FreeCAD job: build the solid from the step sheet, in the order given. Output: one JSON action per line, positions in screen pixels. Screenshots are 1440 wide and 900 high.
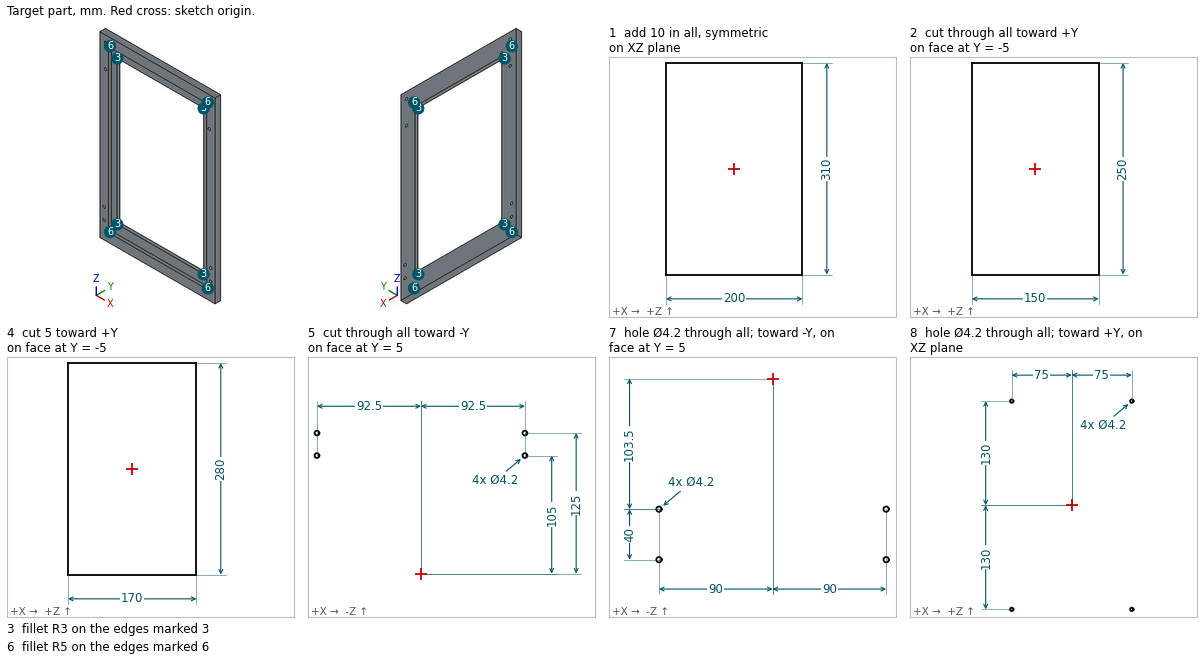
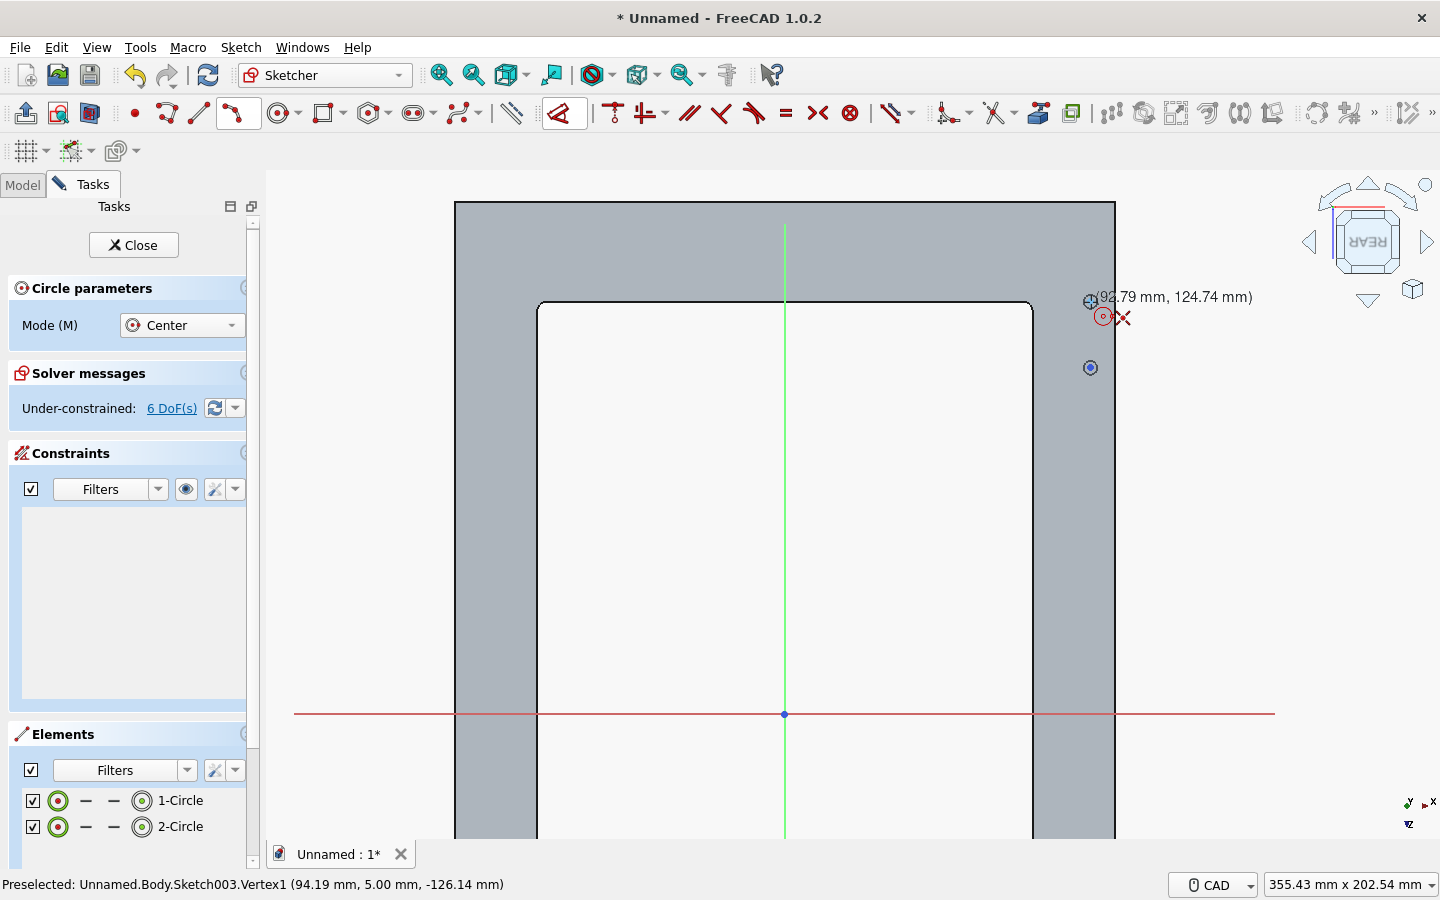
{"action": "scroll", "coordinate": [479, 368], "scroll_direction": "up", "scroll_amount": 6}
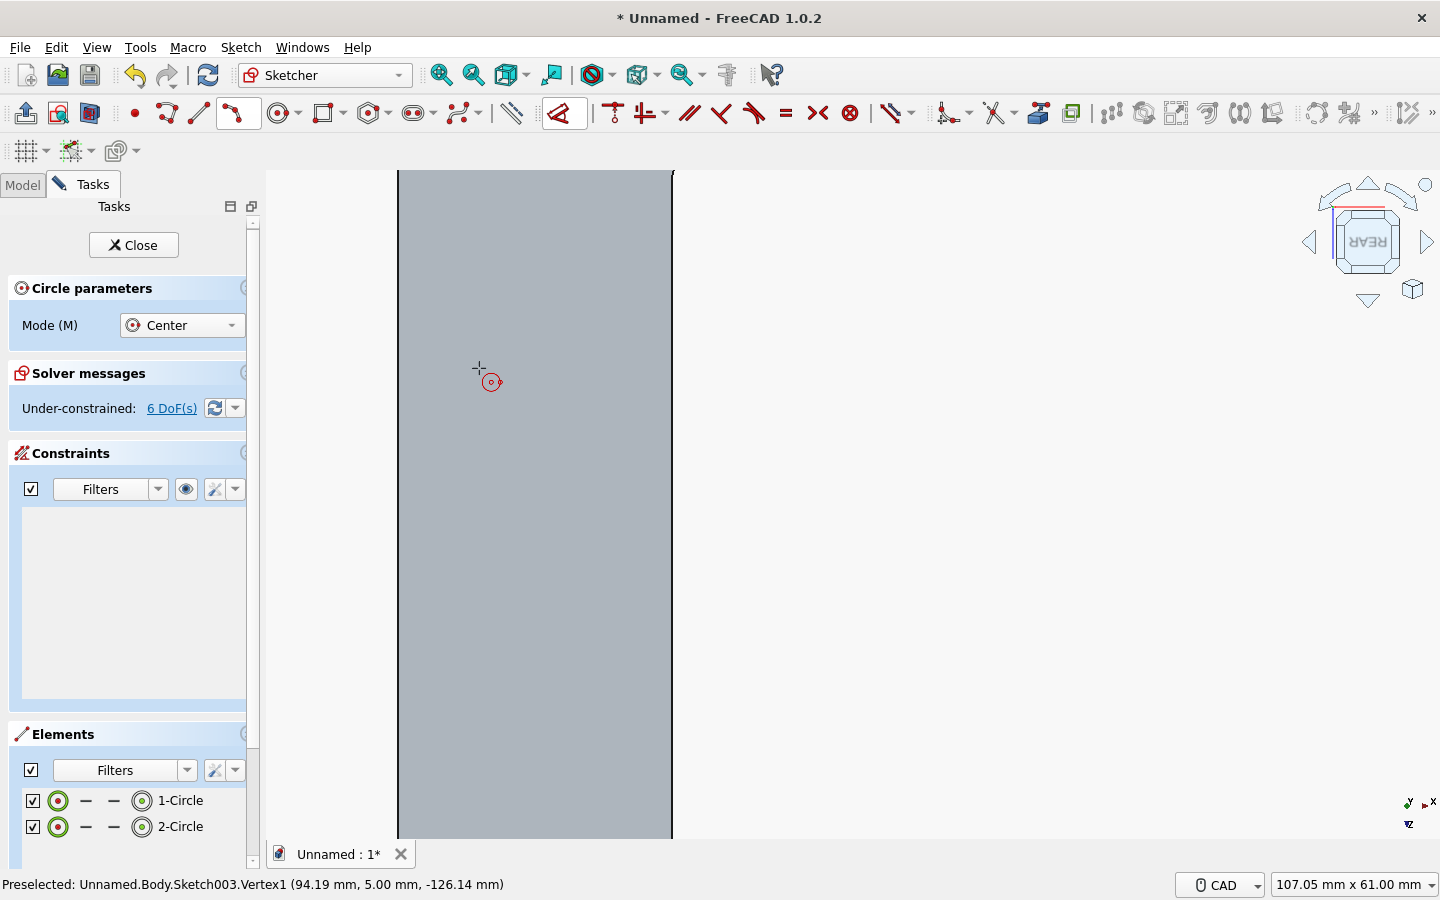
{"action": "left_click", "coordinate": [480, 366]}
{"action": "left_click", "coordinate": [496, 350]}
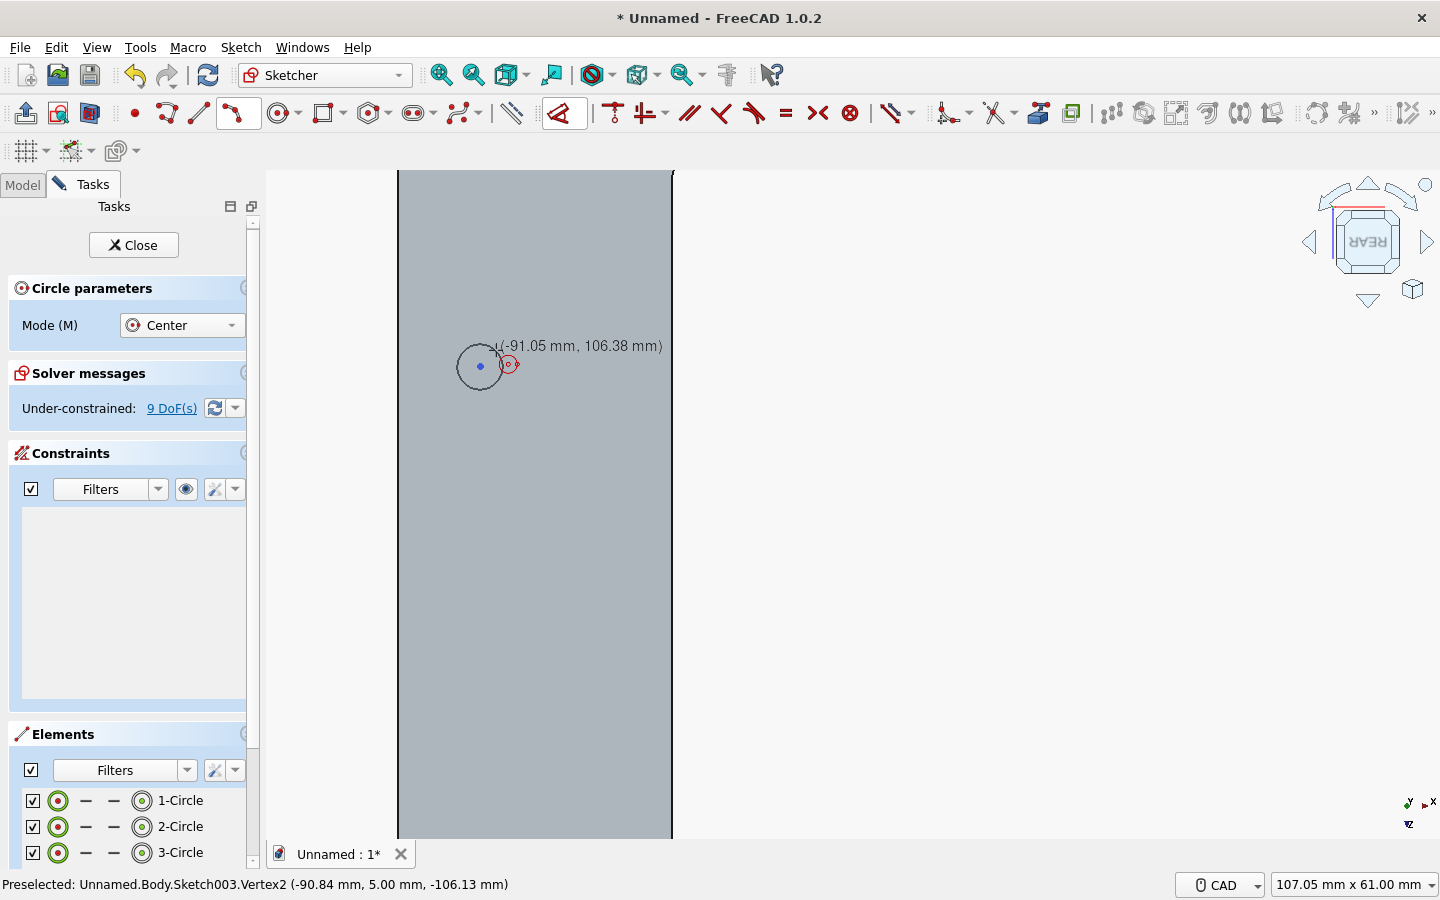
{"action": "scroll", "coordinate": [478, 368], "scroll_direction": "down", "scroll_amount": 6}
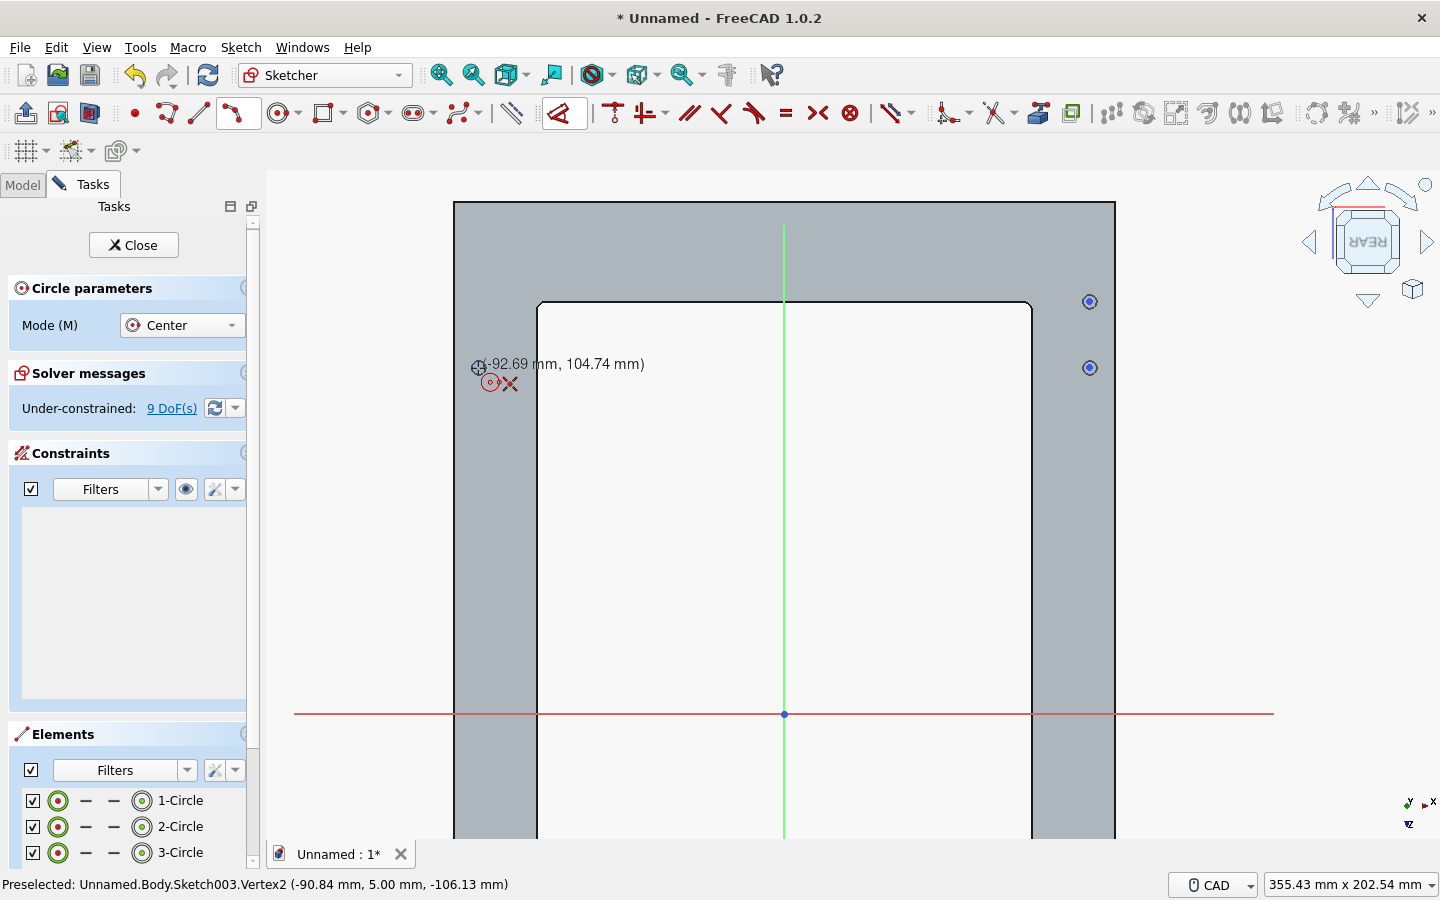
{"action": "scroll", "coordinate": [479, 302], "scroll_direction": "up", "scroll_amount": 6}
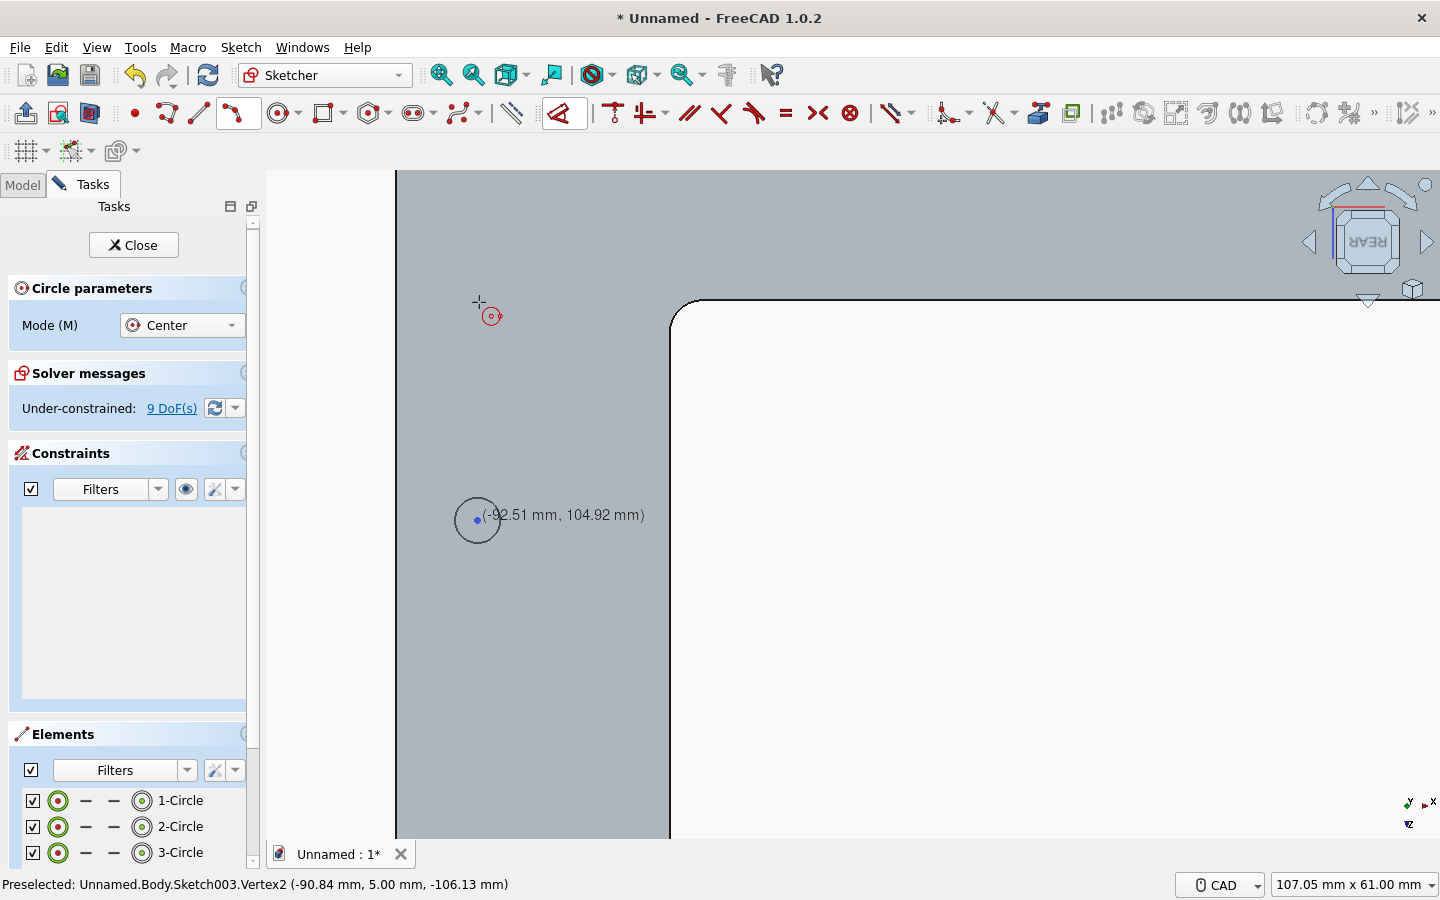
{"action": "left_click", "coordinate": [478, 300]}
{"action": "left_click", "coordinate": [494, 284]}
{"action": "key", "text": "Escape"}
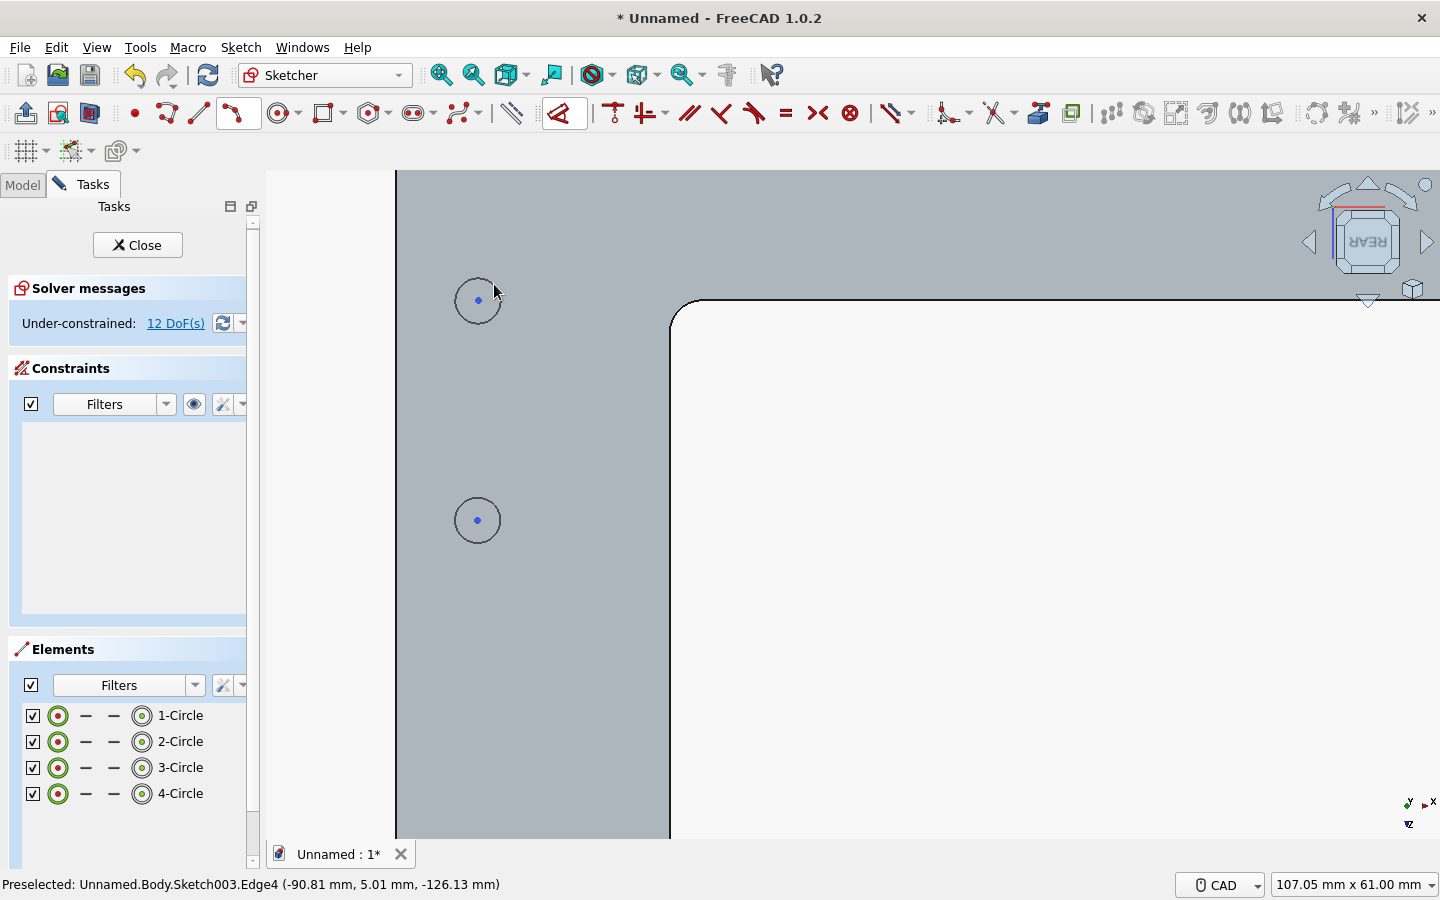
{"action": "scroll", "coordinate": [479, 302], "scroll_direction": "down", "scroll_amount": 6}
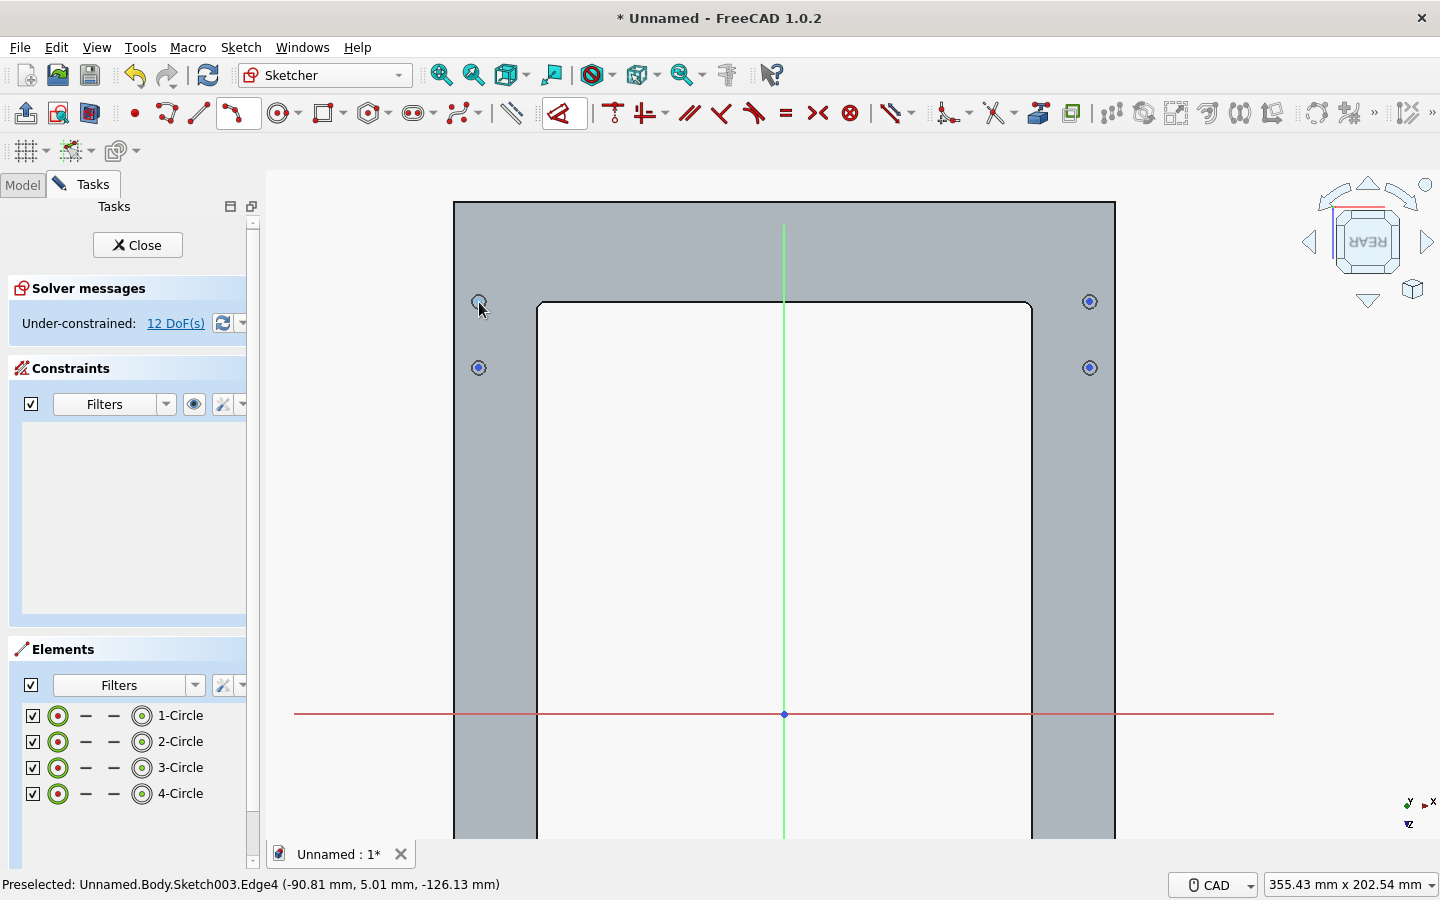
{"action": "scroll", "coordinate": [1095, 363], "scroll_direction": "up", "scroll_amount": 4}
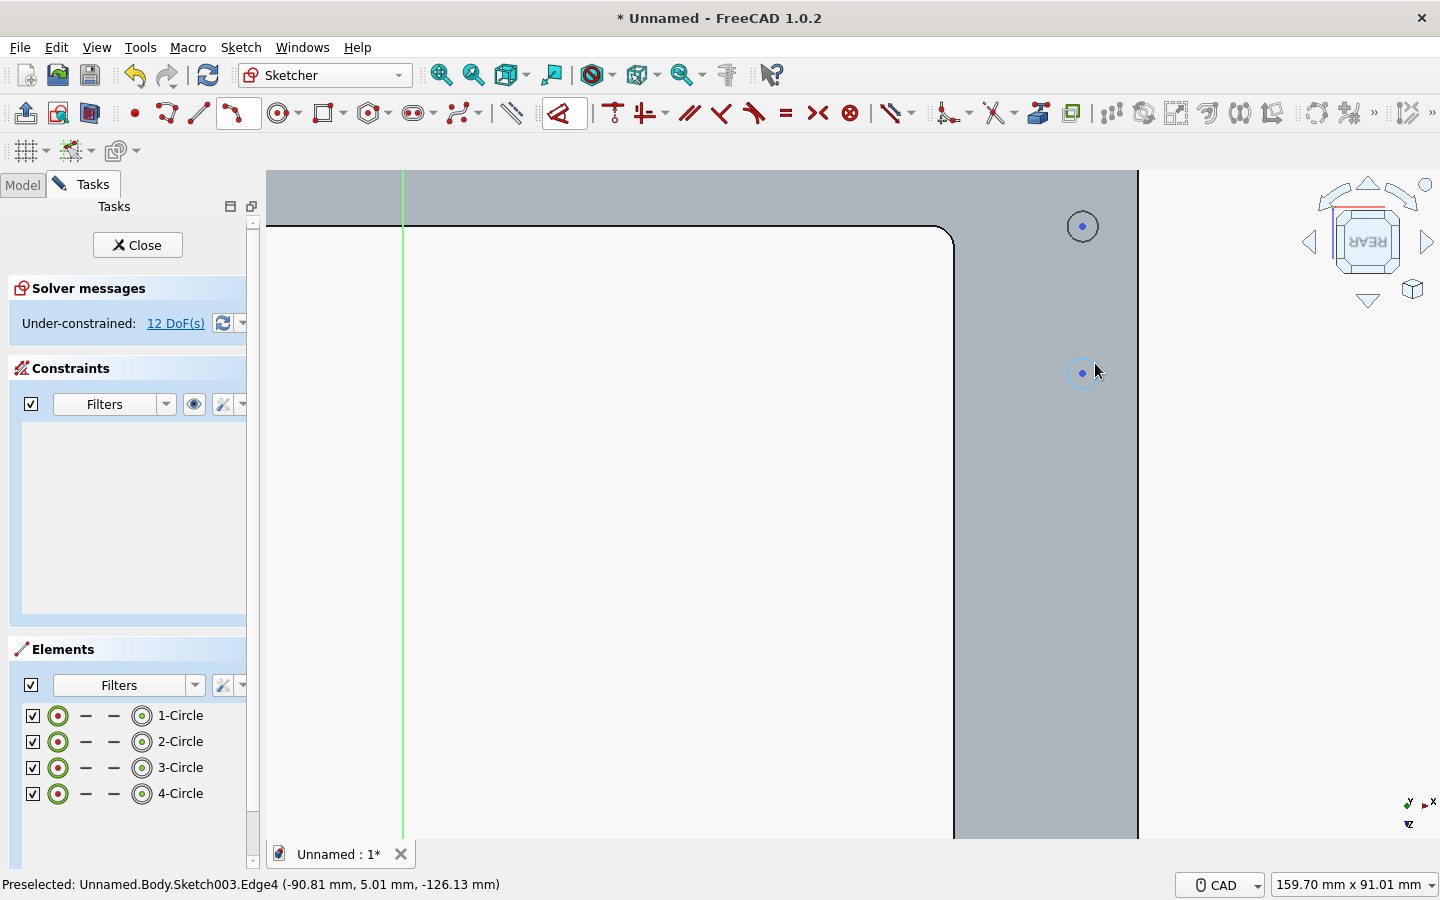
{"action": "left_click", "coordinate": [1093, 363]}